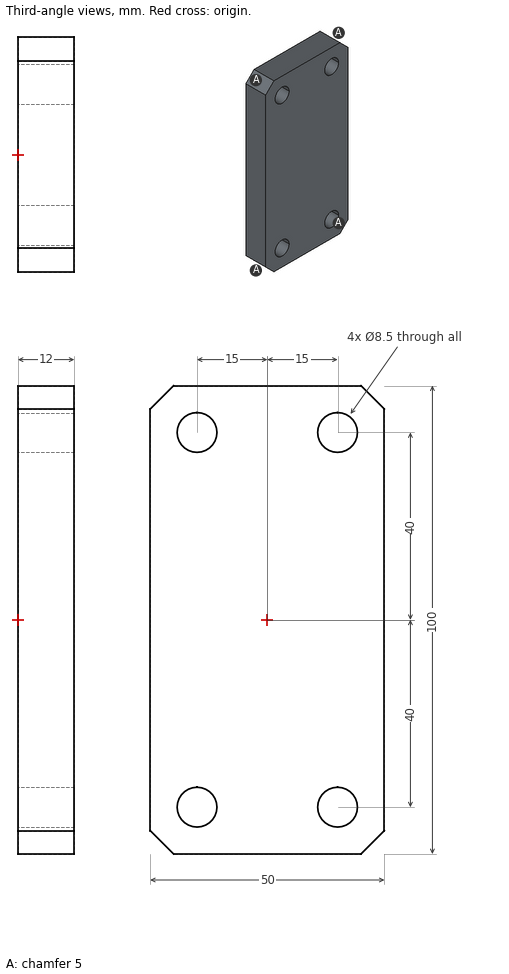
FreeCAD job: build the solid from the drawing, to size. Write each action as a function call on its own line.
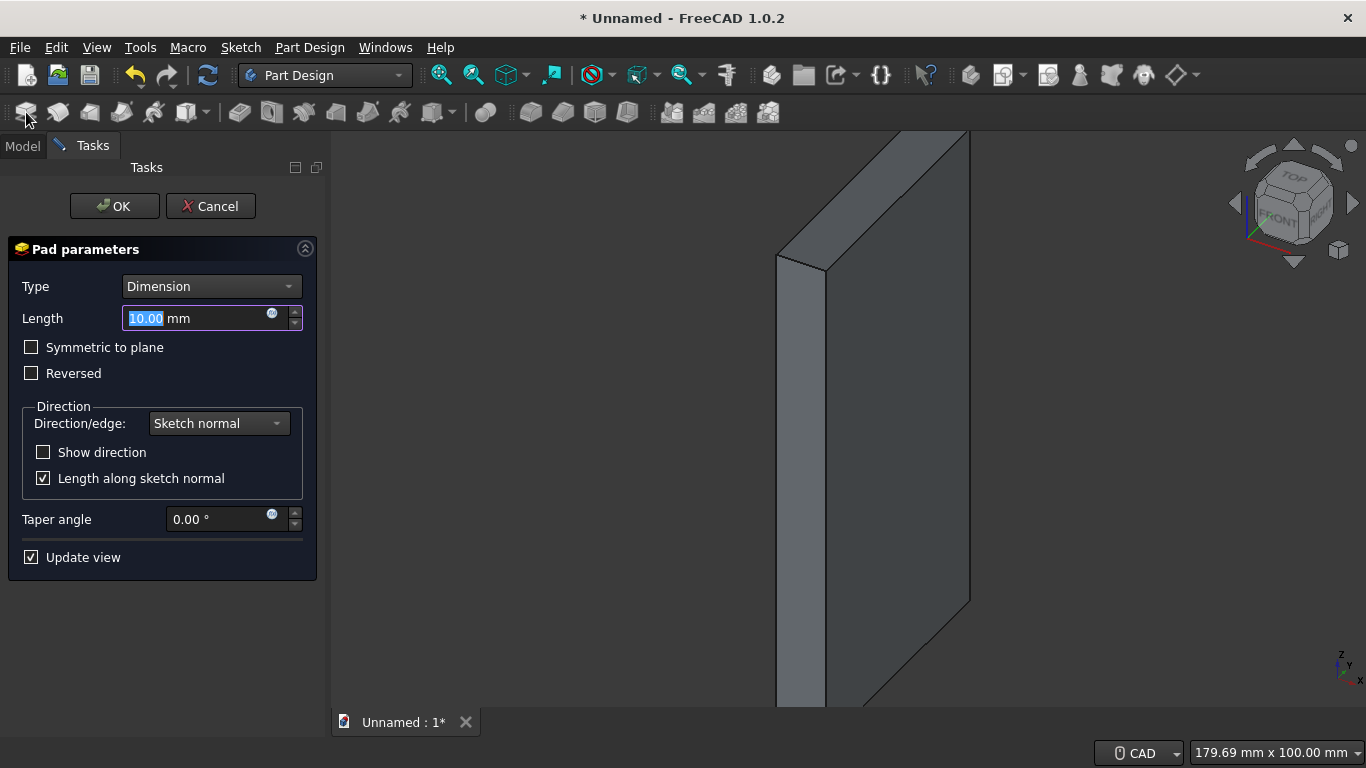
text(12)
key(Tab)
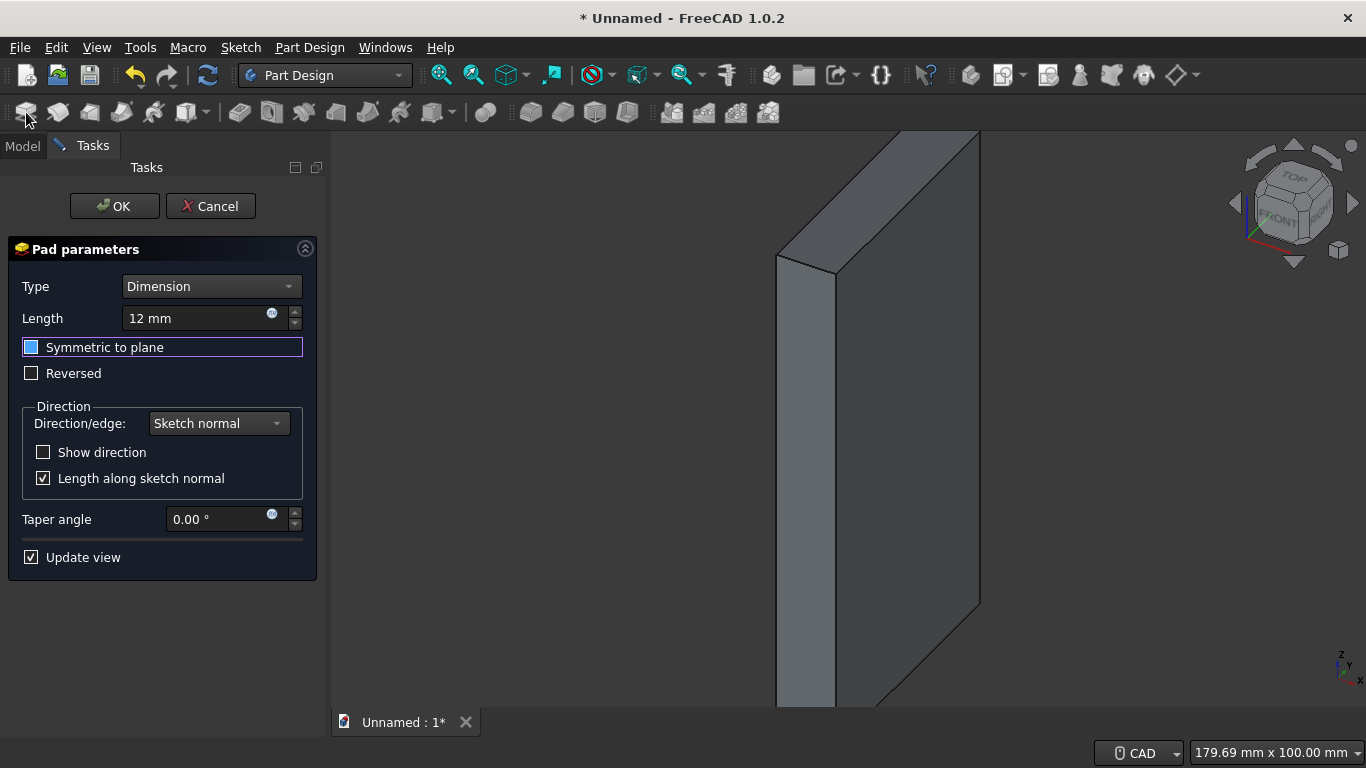
click(115, 206)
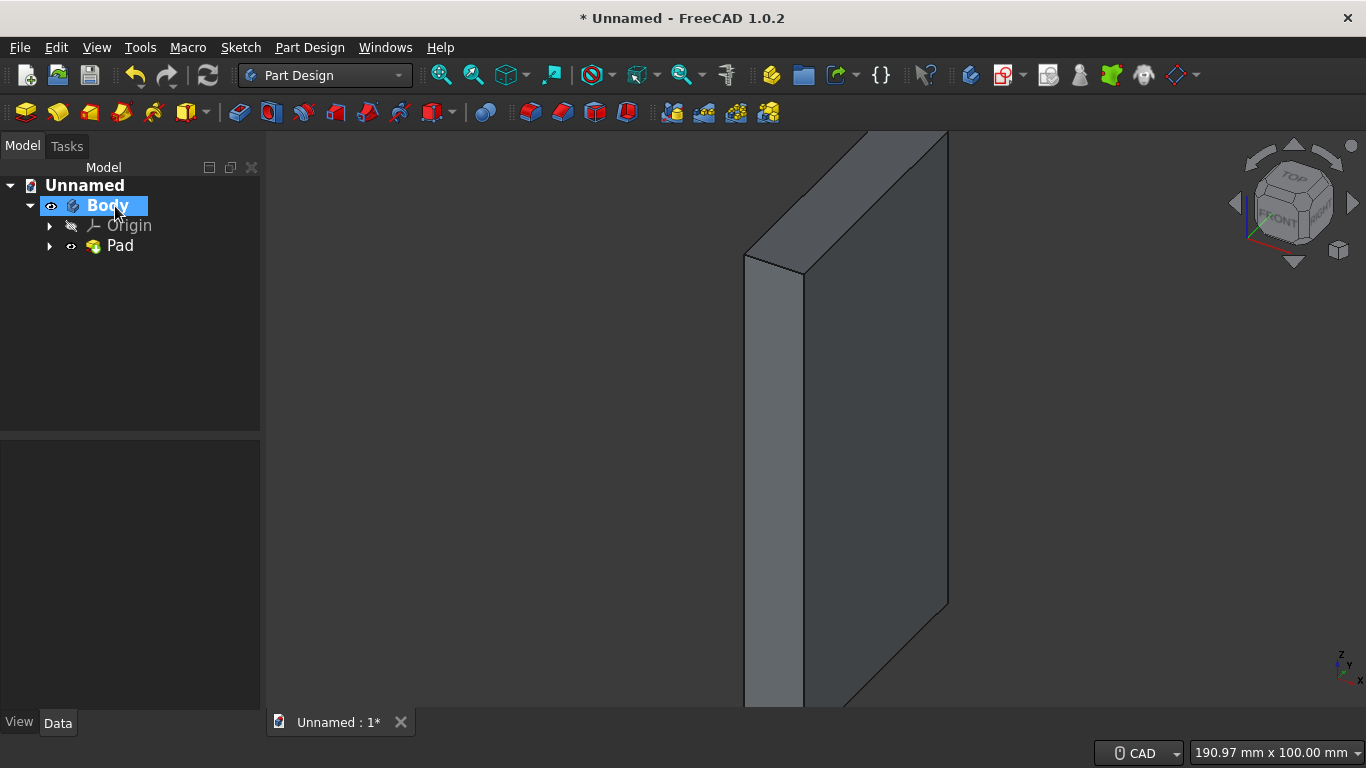
click(442, 76)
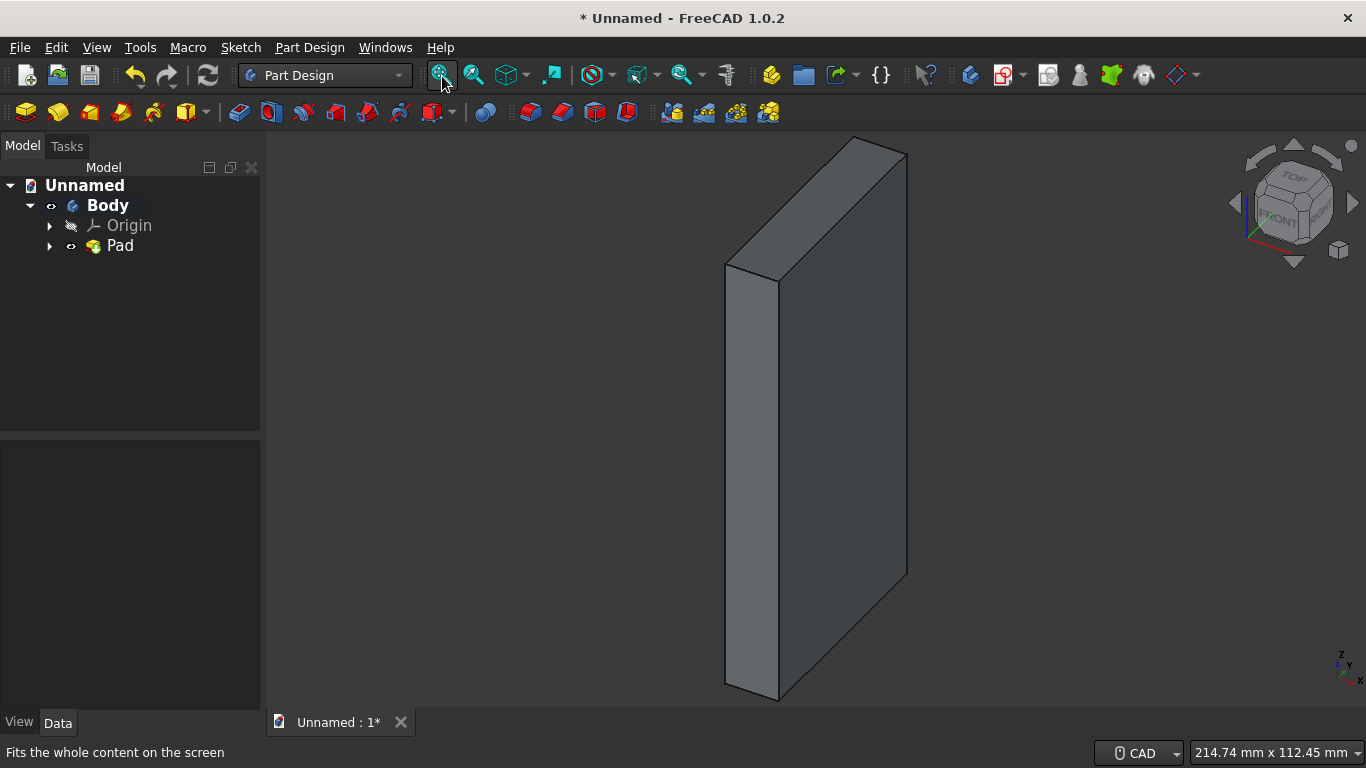
click(843, 427)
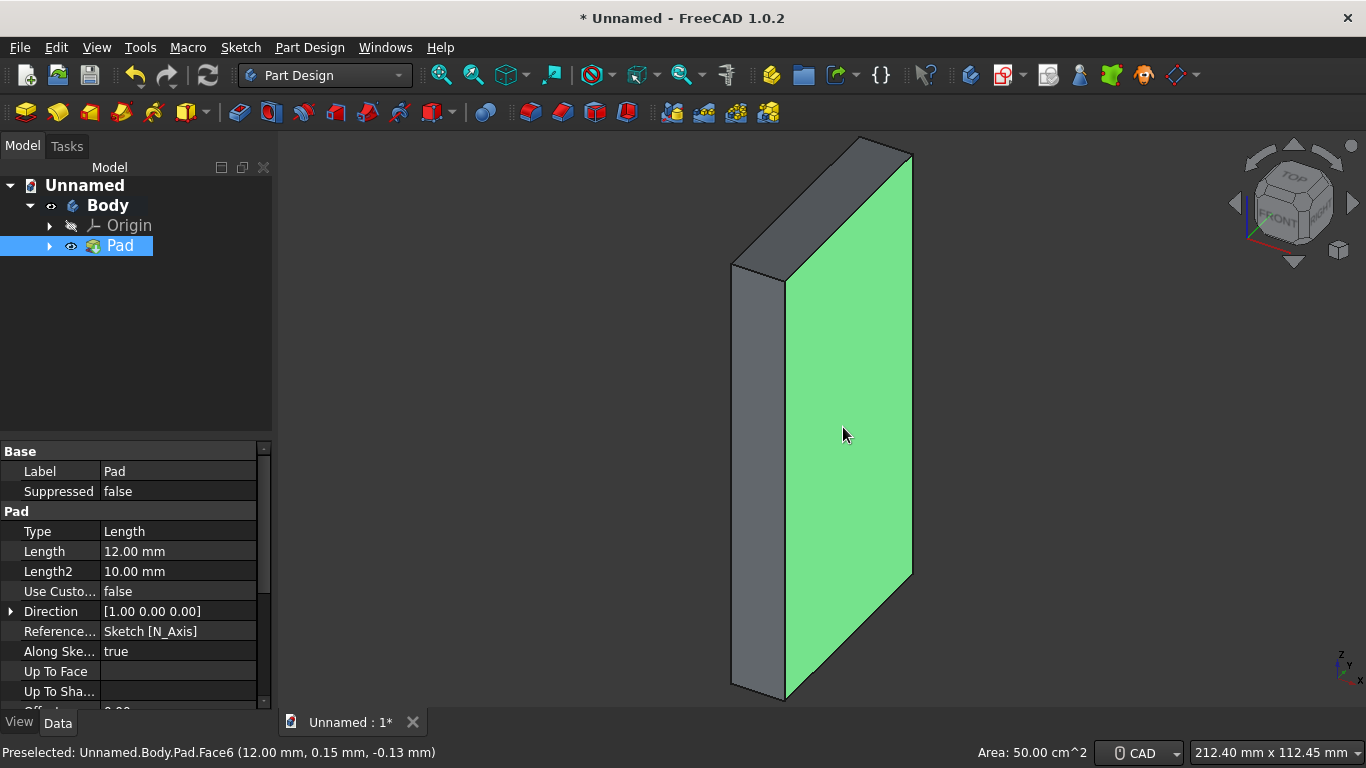
click(1004, 76)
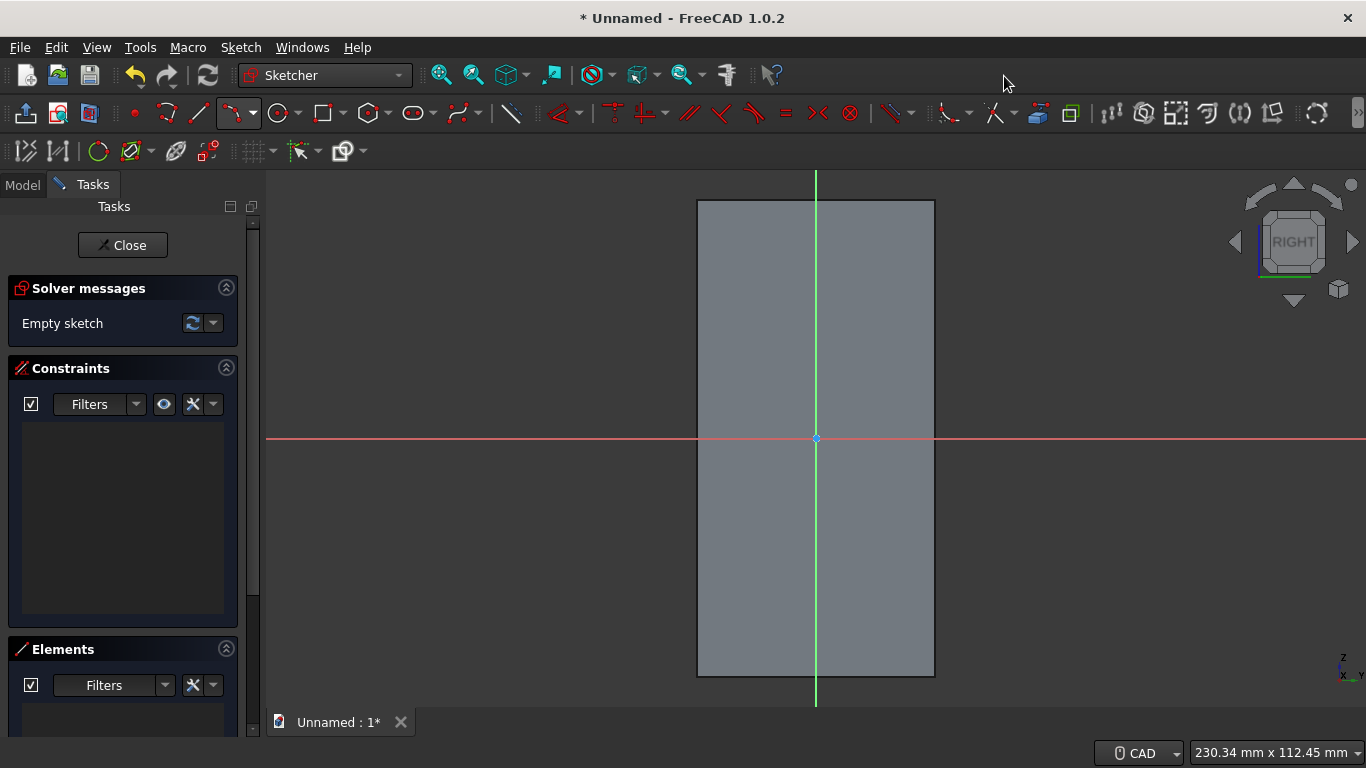
click(278, 114)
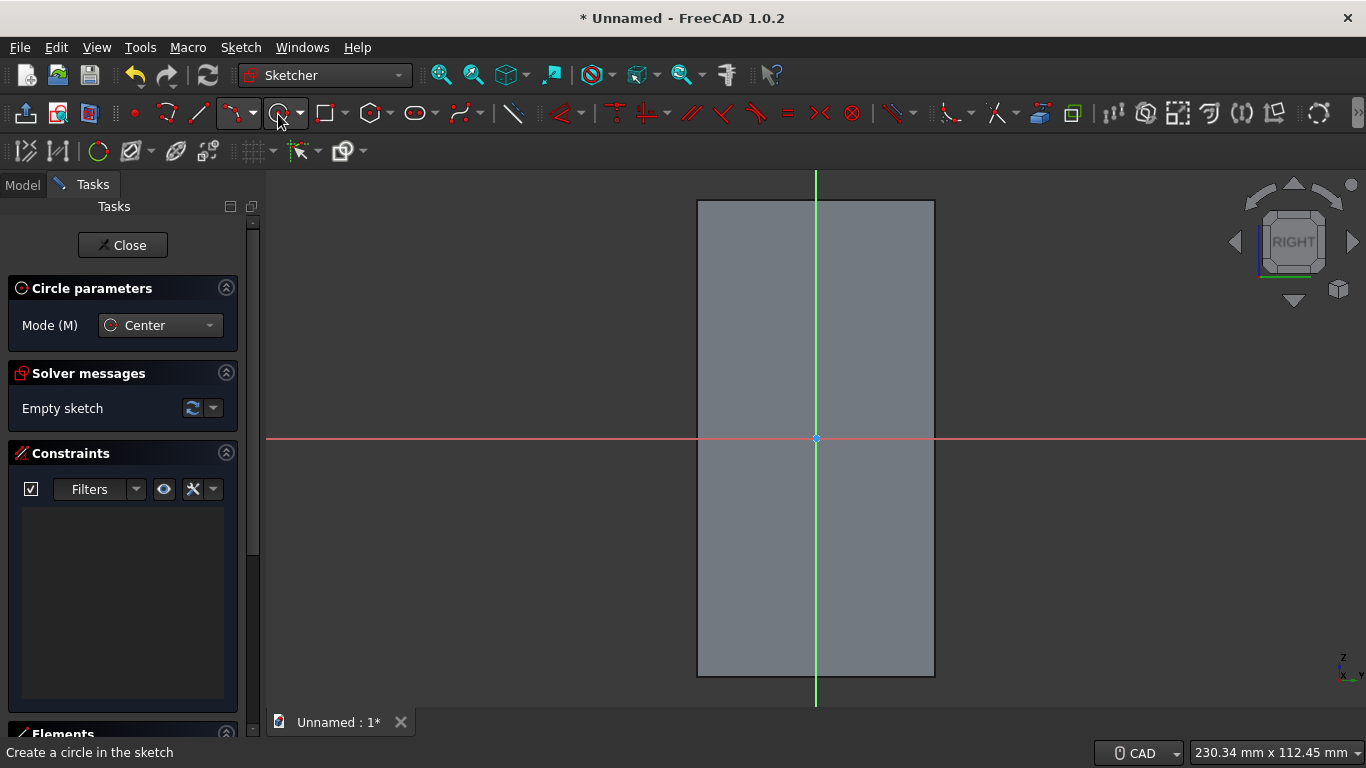
click(888, 247)
move(902, 233)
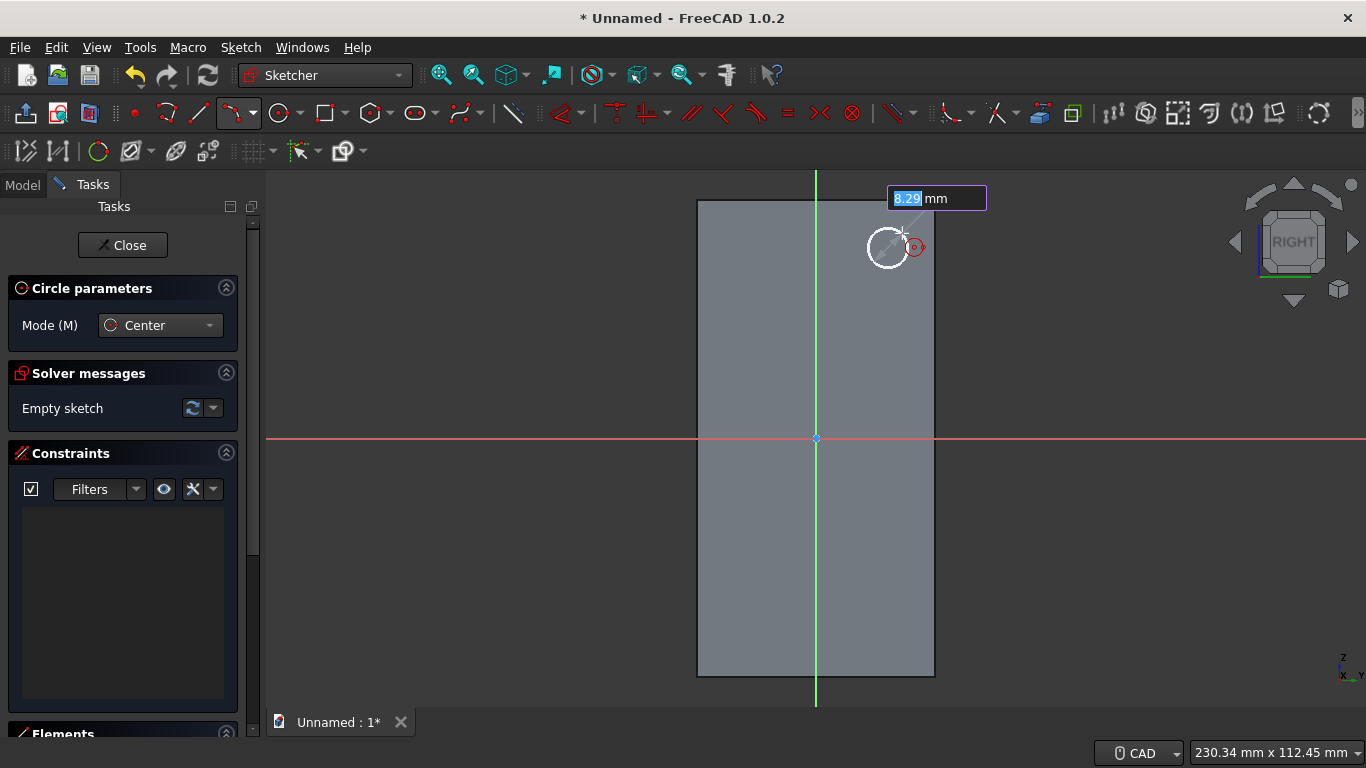
text(8.5)
key(Return)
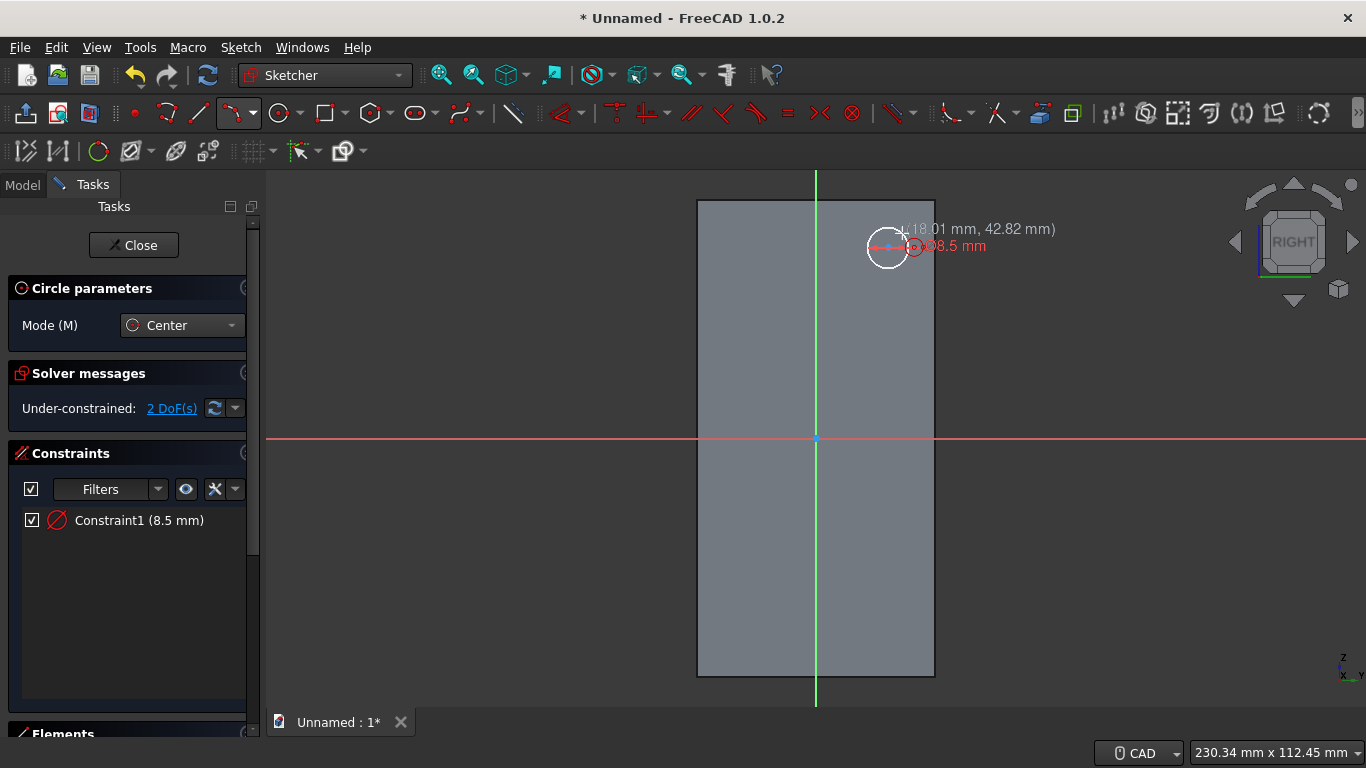
click(744, 247)
move(759, 233)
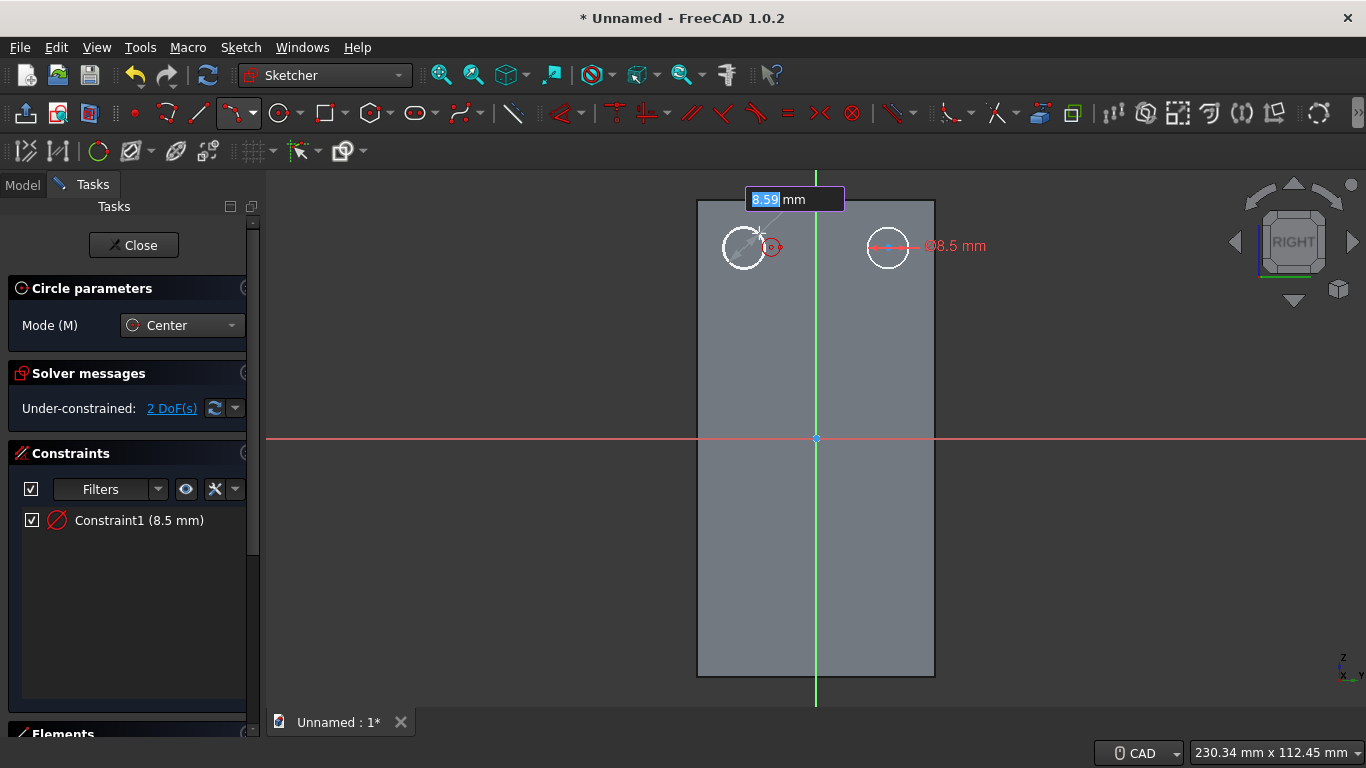
text(8.5)
key(Return)